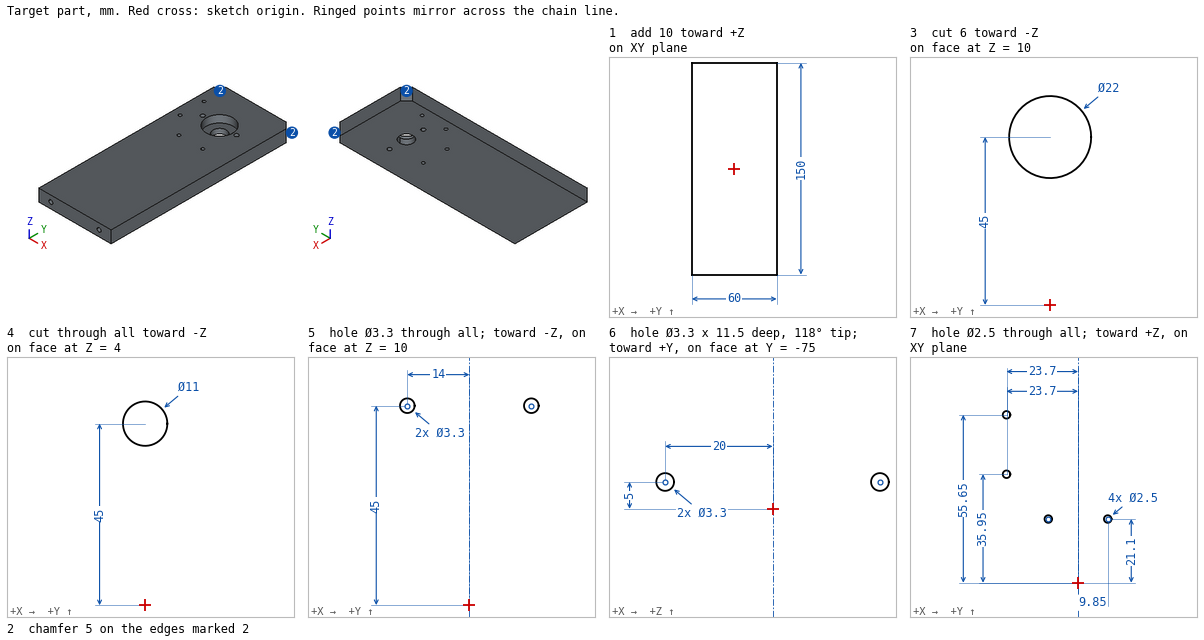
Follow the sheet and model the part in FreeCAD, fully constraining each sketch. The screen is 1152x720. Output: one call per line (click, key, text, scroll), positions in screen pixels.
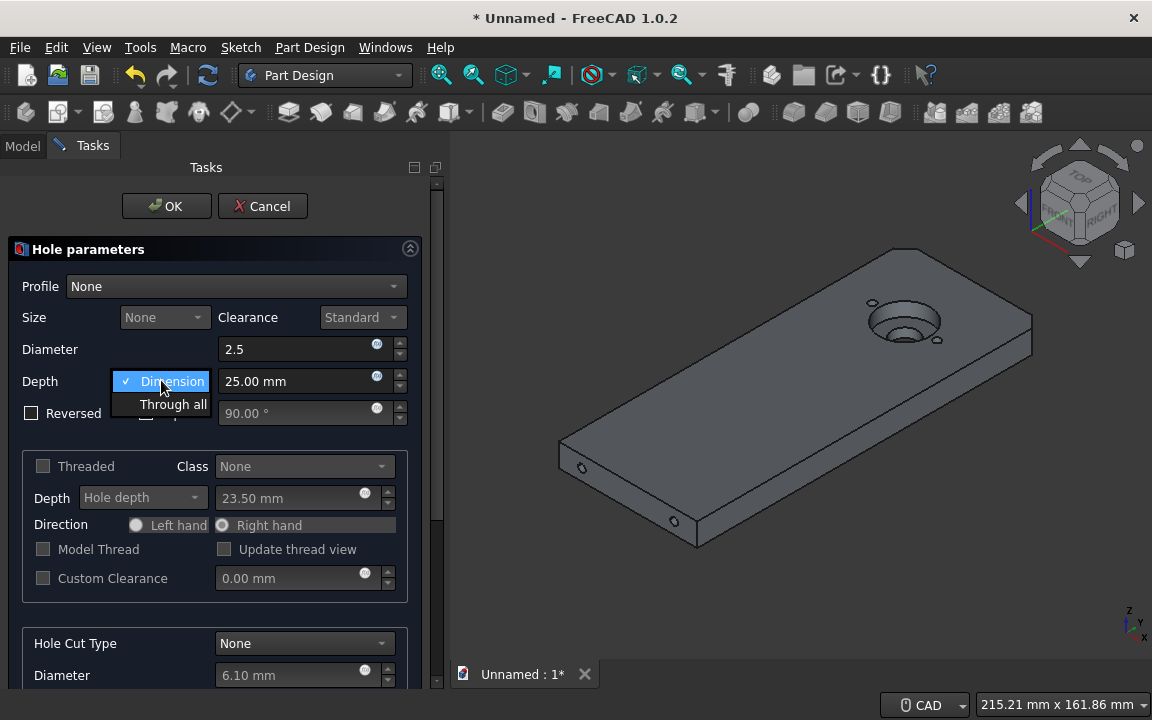
click(160, 404)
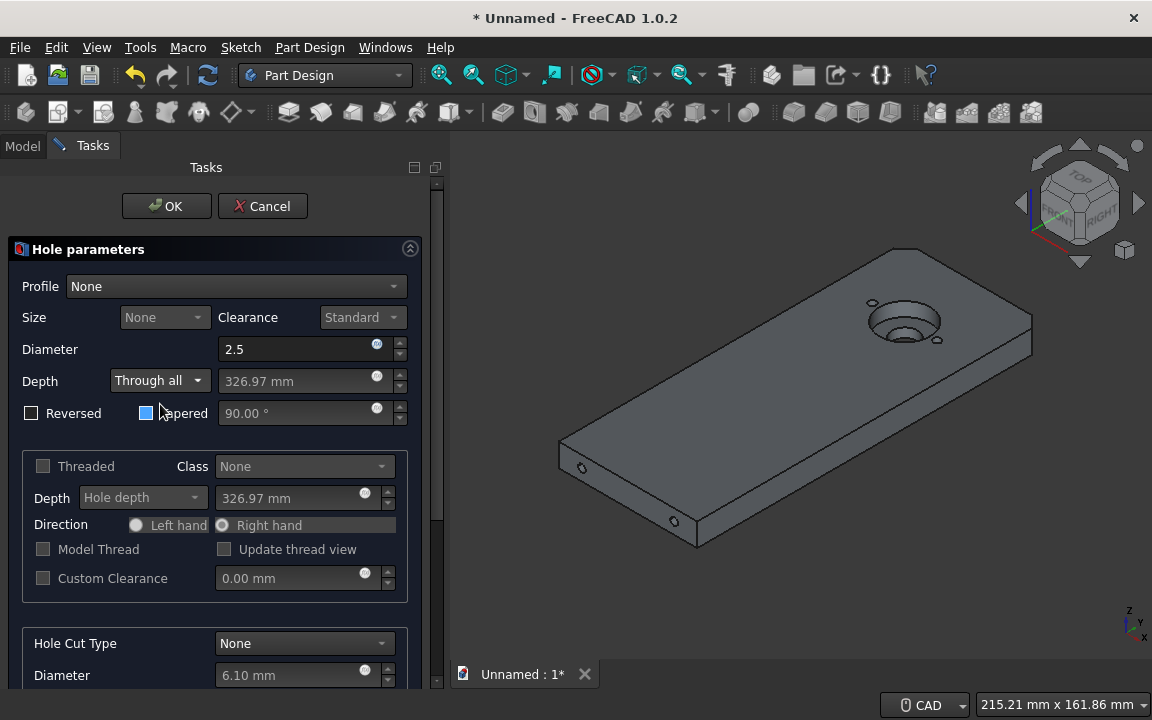
click(30, 413)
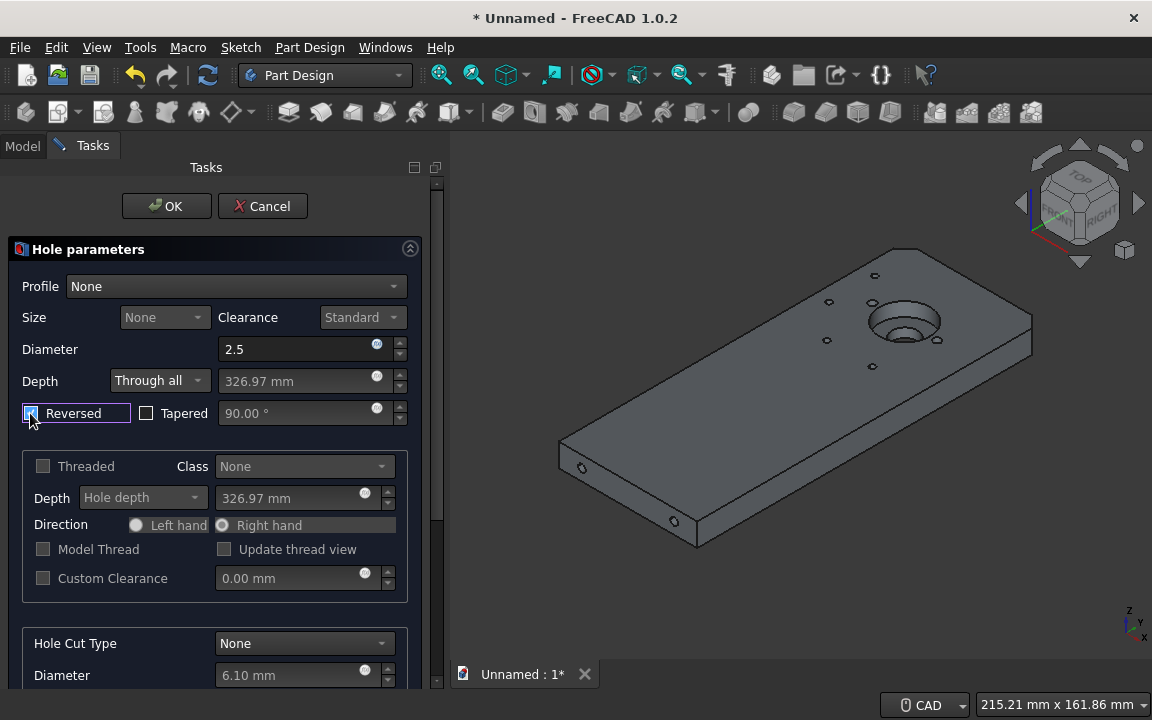
click(167, 206)